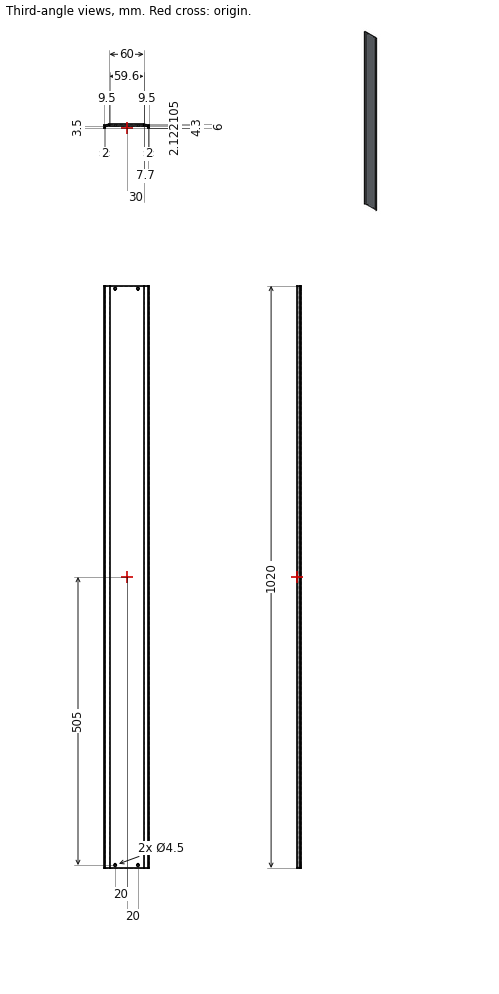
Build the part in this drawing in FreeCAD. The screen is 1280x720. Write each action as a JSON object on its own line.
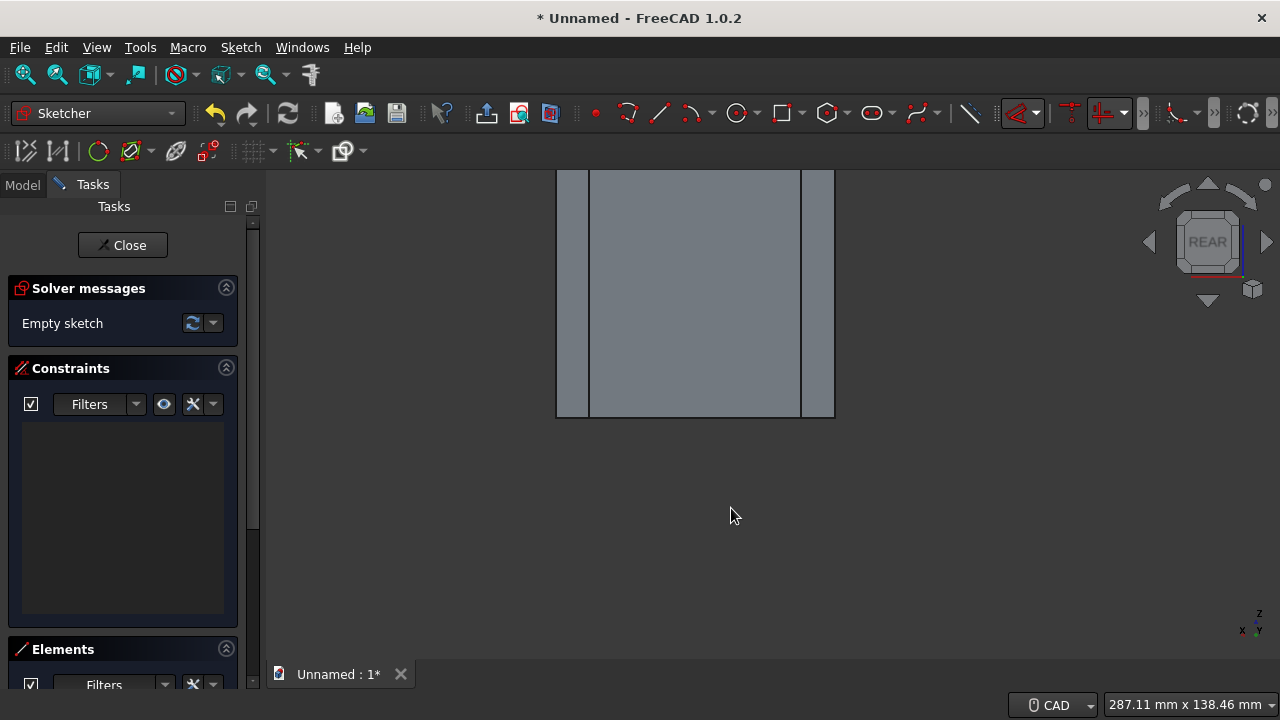
{"action": "scroll", "coordinate": [692, 396], "scroll_direction": "up", "scroll_amount": 7}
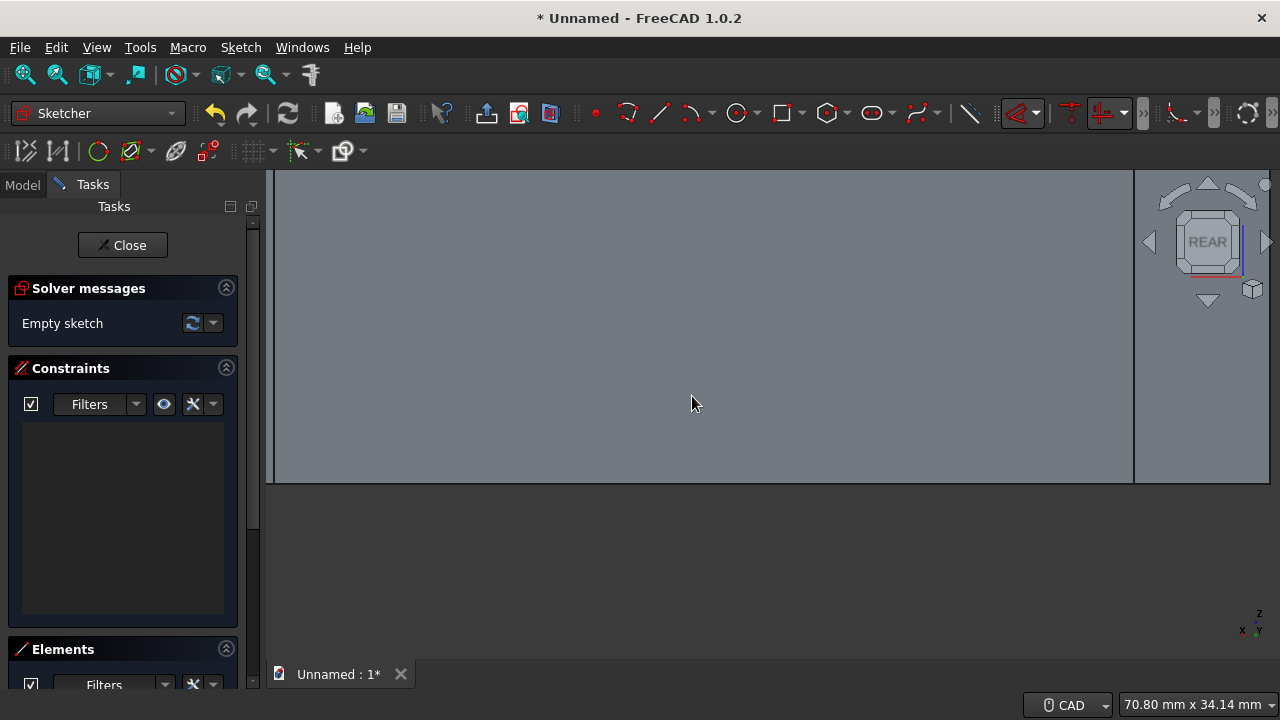
{"action": "left_click", "coordinate": [738, 114]}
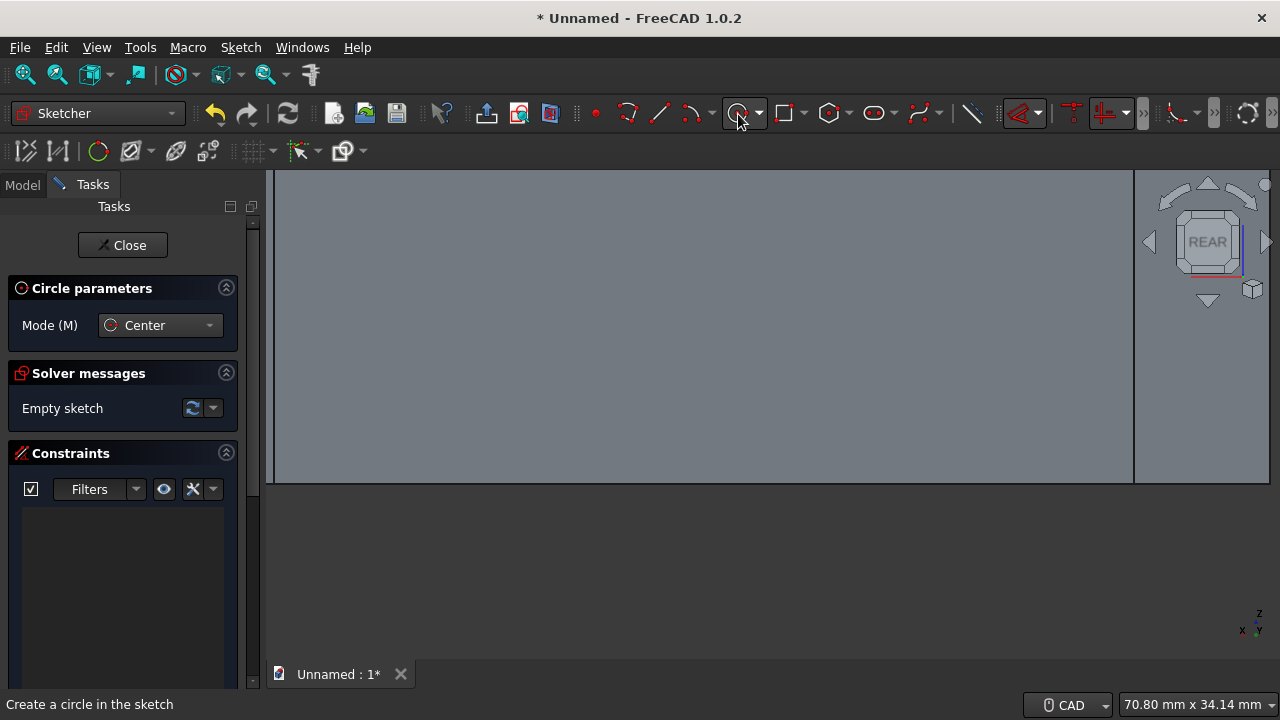
{"action": "left_click", "coordinate": [990, 412]}
{"action": "mouse_move", "coordinate": [1013, 389]}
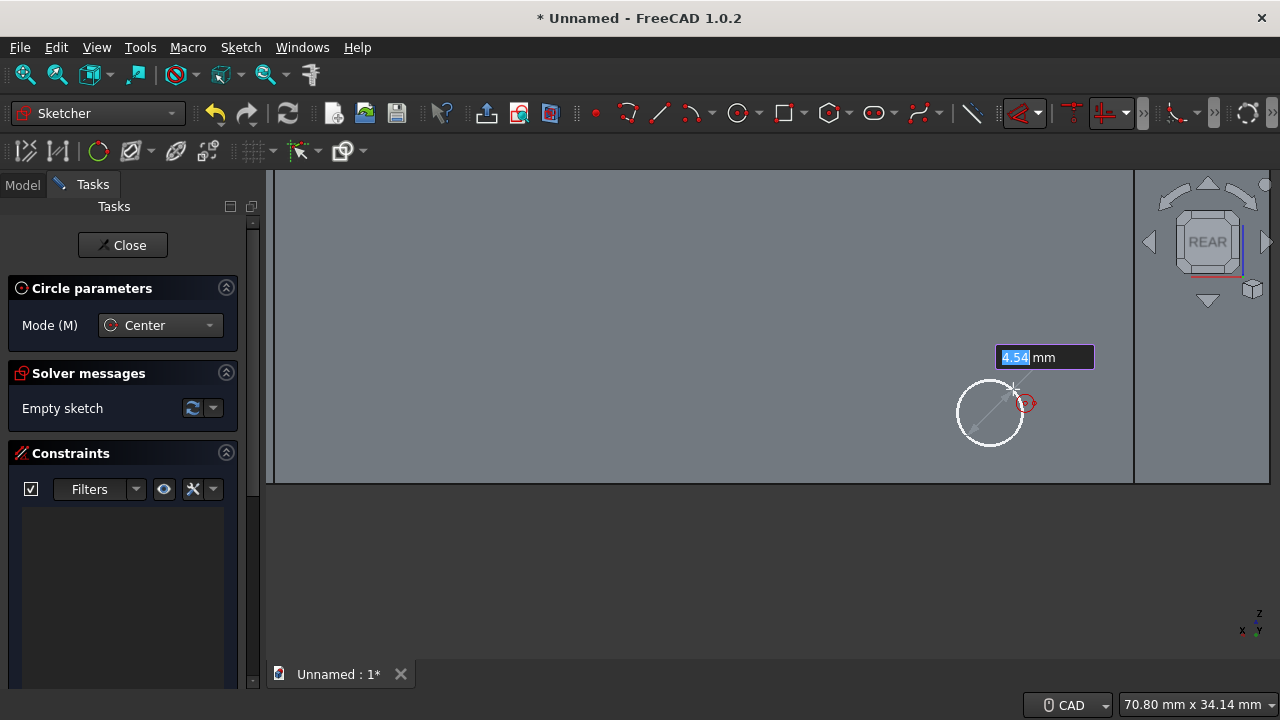
{"action": "type", "text": "4.5"}
{"action": "key", "text": "Return"}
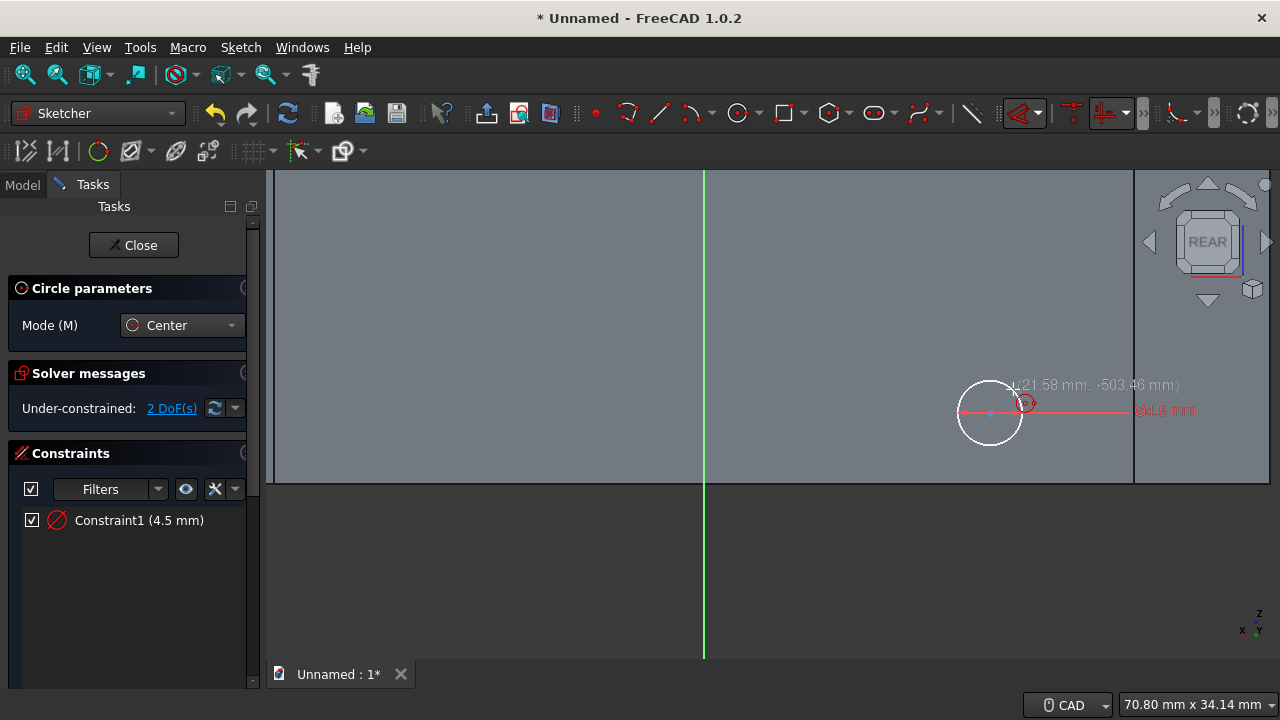
{"action": "left_click", "coordinate": [418, 412]}
{"action": "mouse_move", "coordinate": [440, 389]}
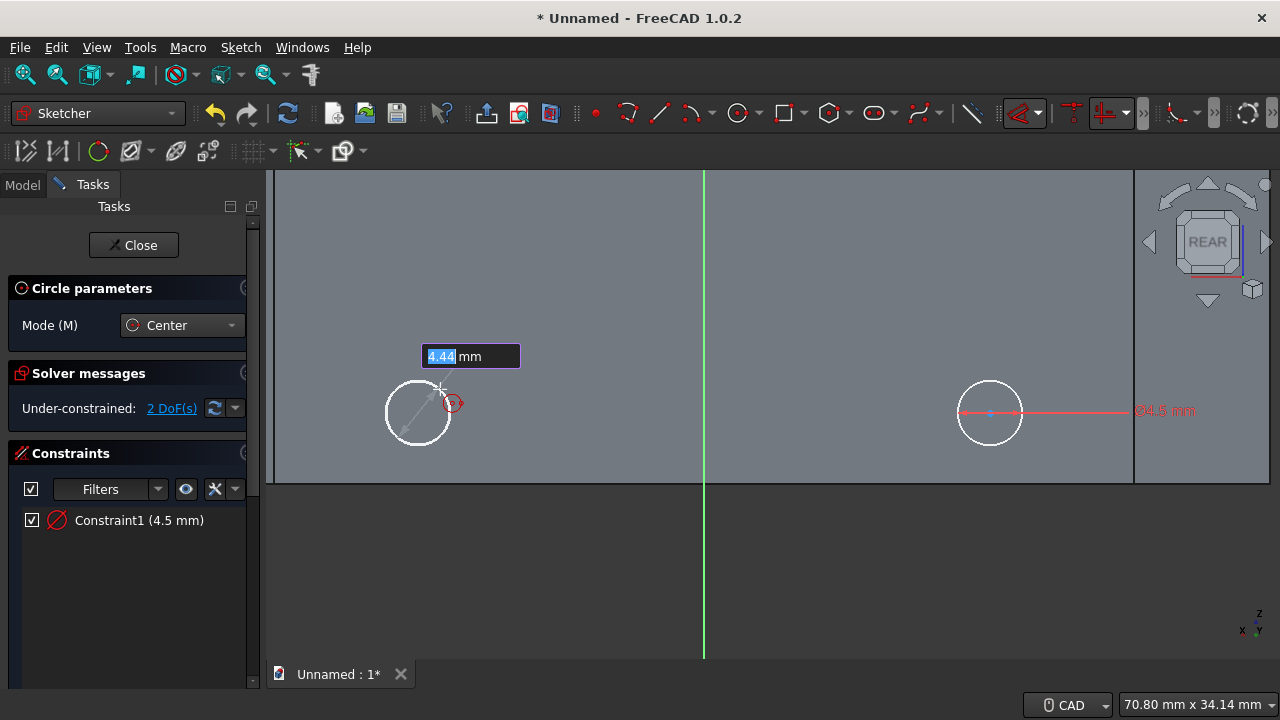
{"action": "type", "text": "4.5"}
{"action": "key", "text": "Return"}
{"action": "key", "text": "Escape"}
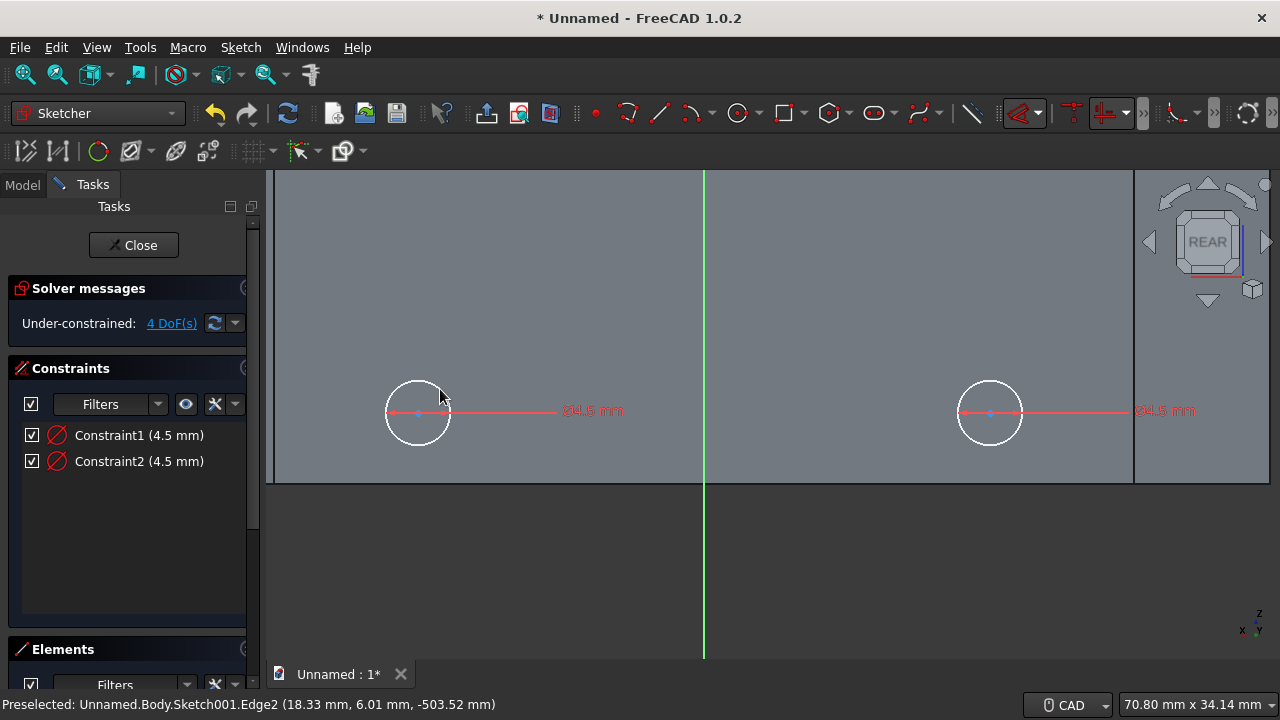
{"action": "left_click", "coordinate": [990, 413]}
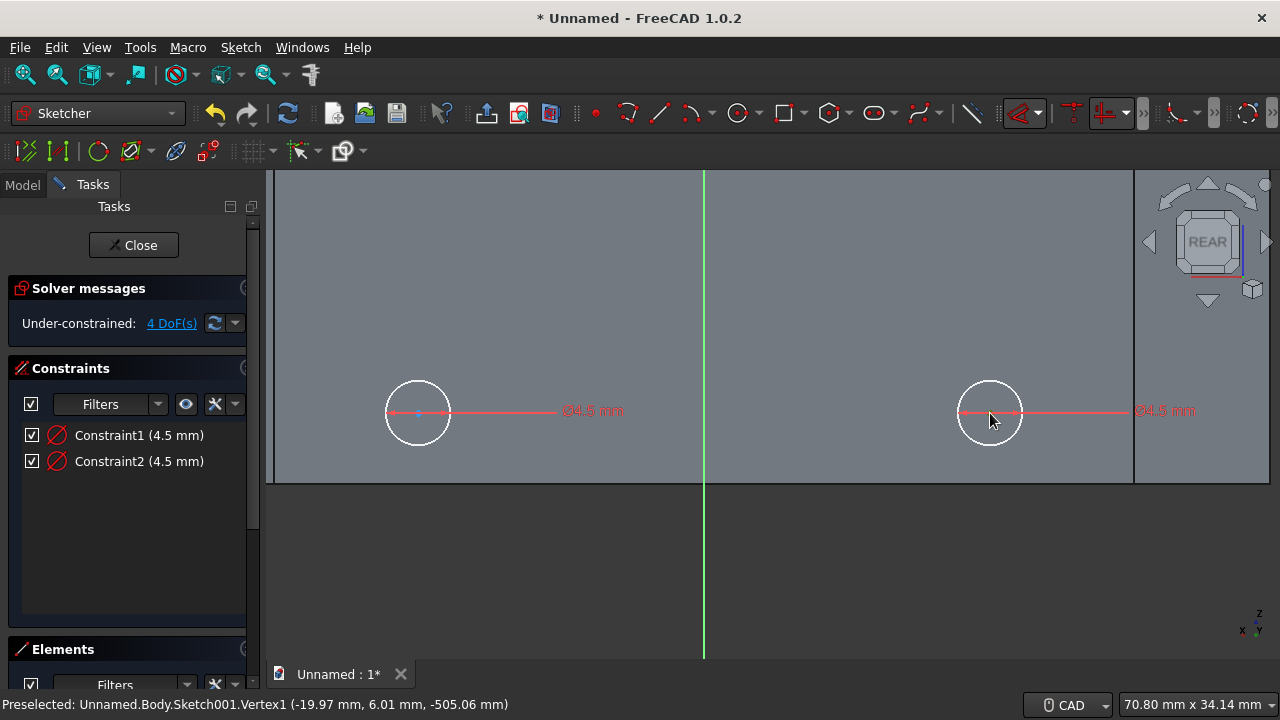
{"action": "key", "text": "l"}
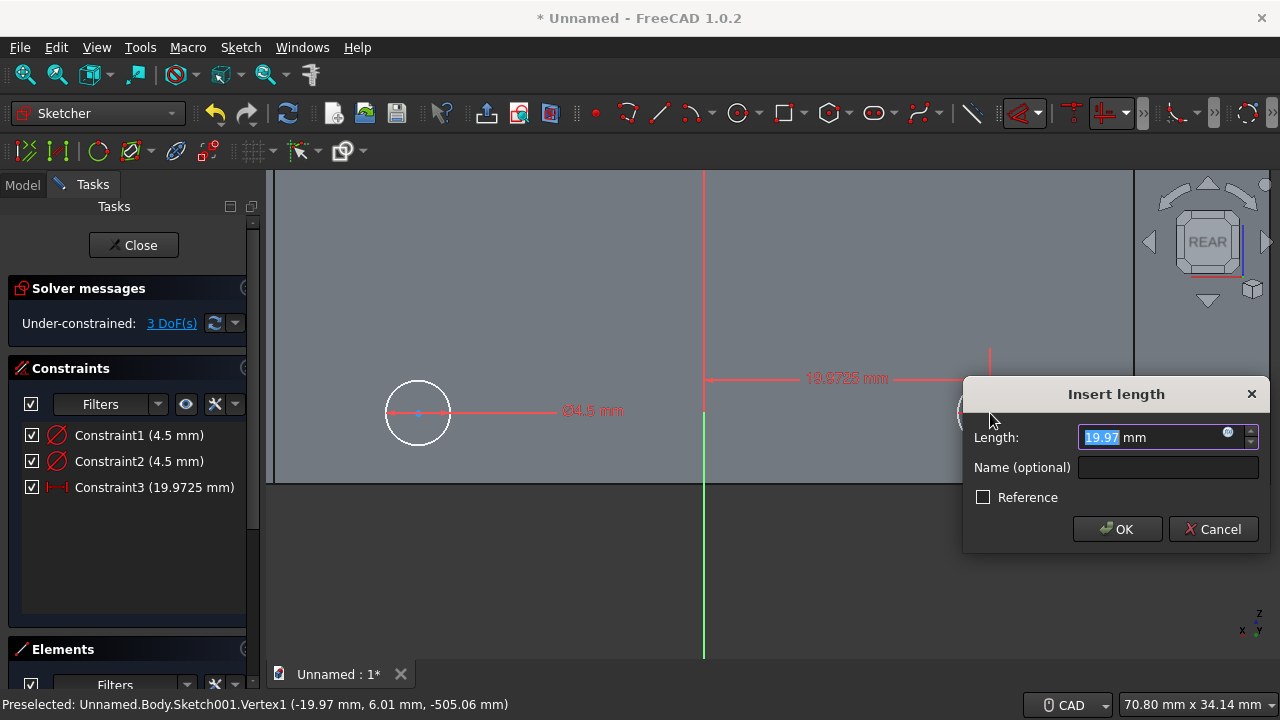
{"action": "type", "text": "20"}
{"action": "key", "text": "Return"}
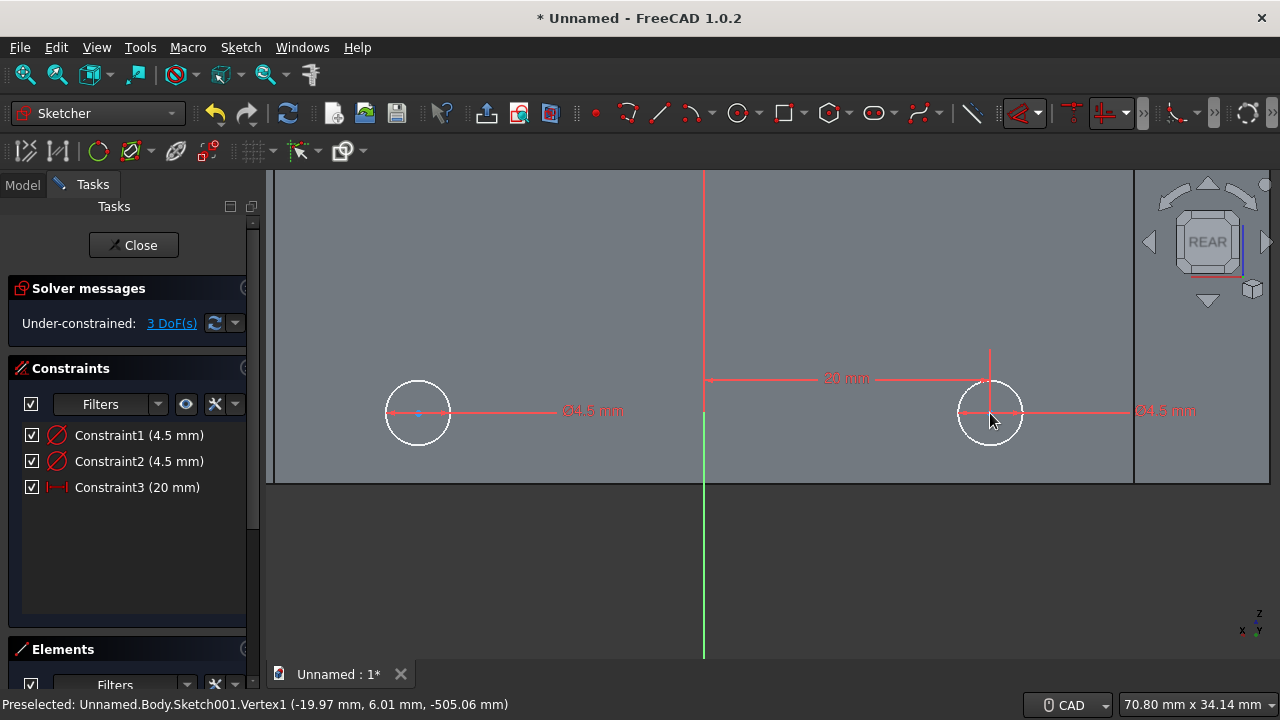
{"action": "left_click", "coordinate": [418, 413]}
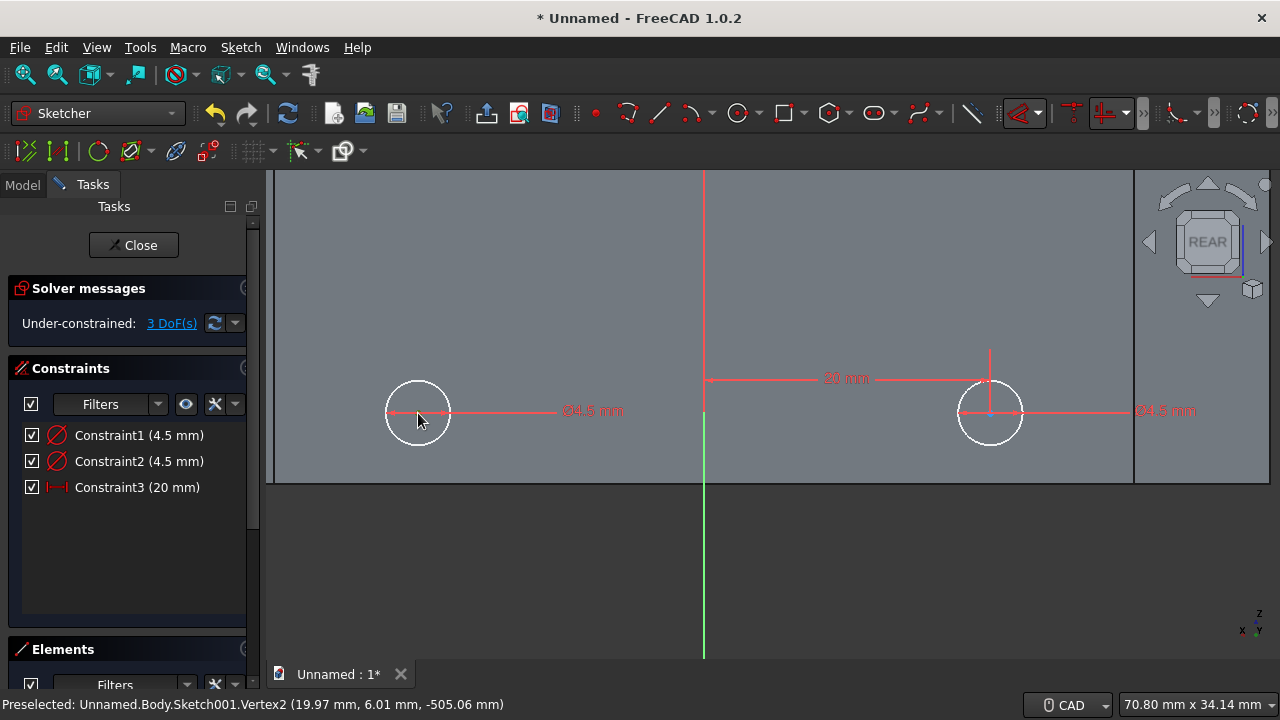
{"action": "key", "text": "l"}